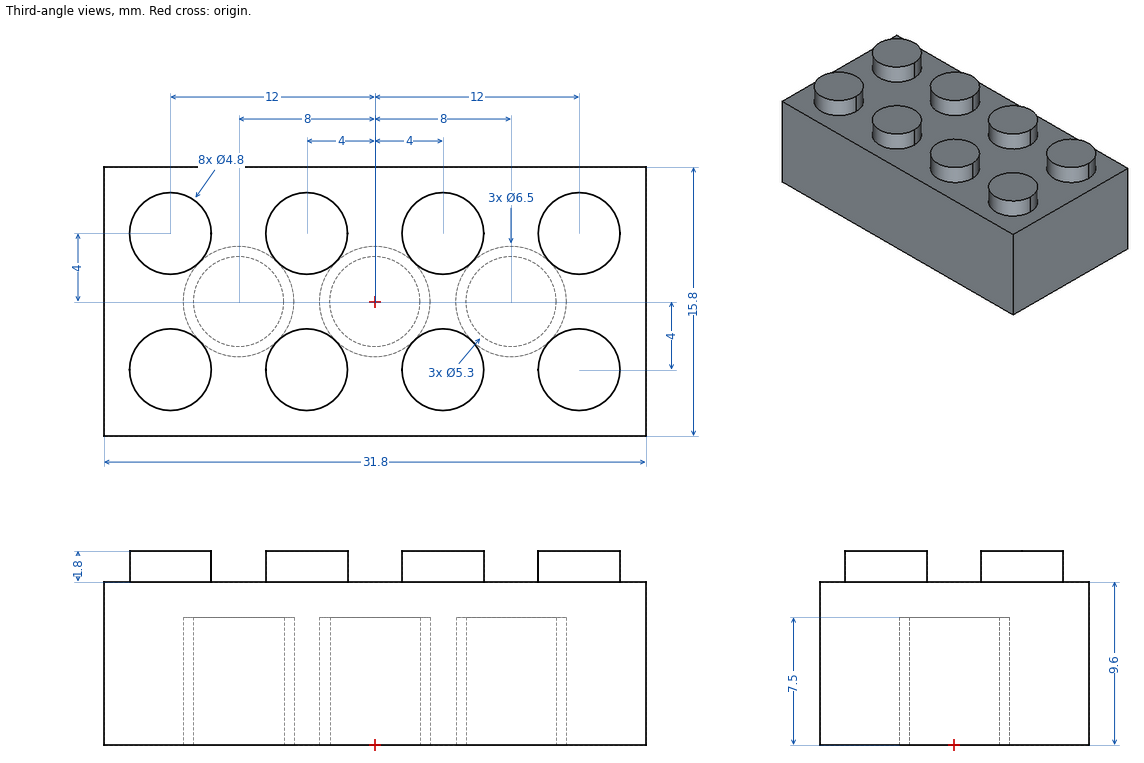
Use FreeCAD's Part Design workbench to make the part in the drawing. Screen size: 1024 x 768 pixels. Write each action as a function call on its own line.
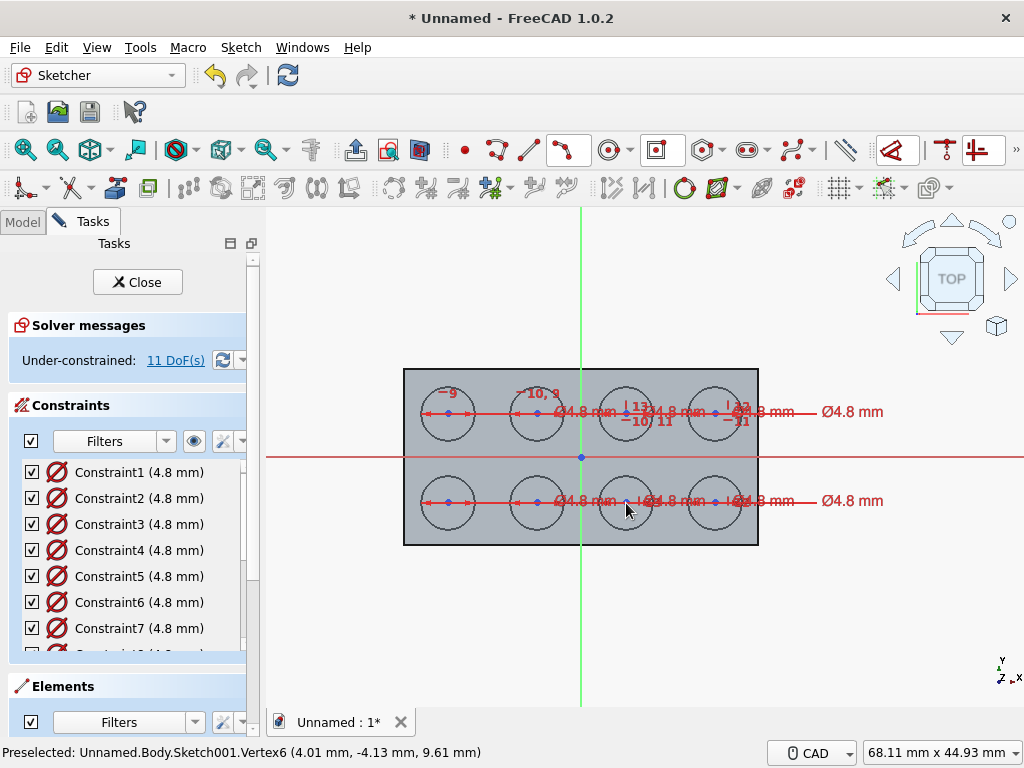
click(715, 503)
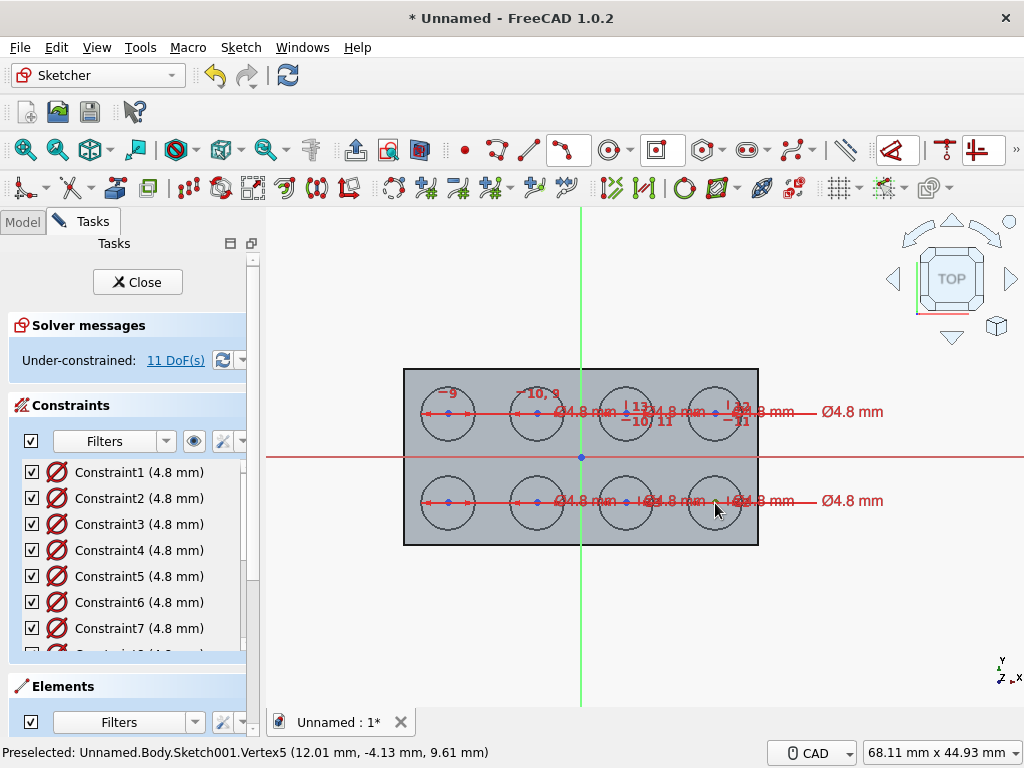
click(626, 503)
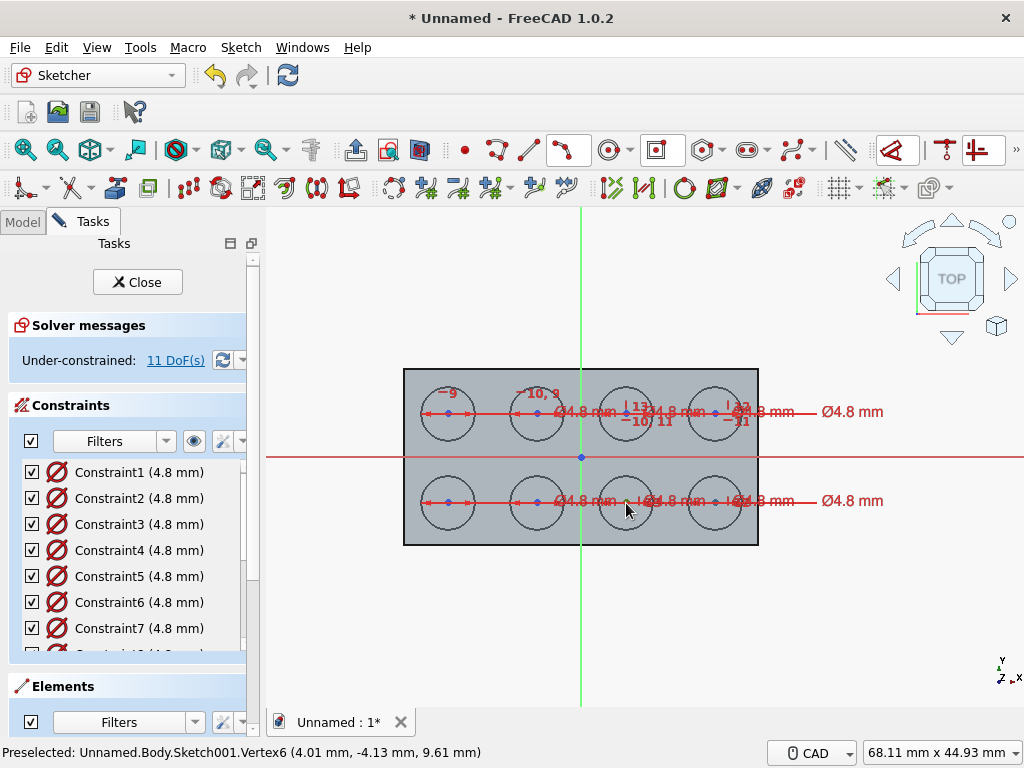
click(1000, 150)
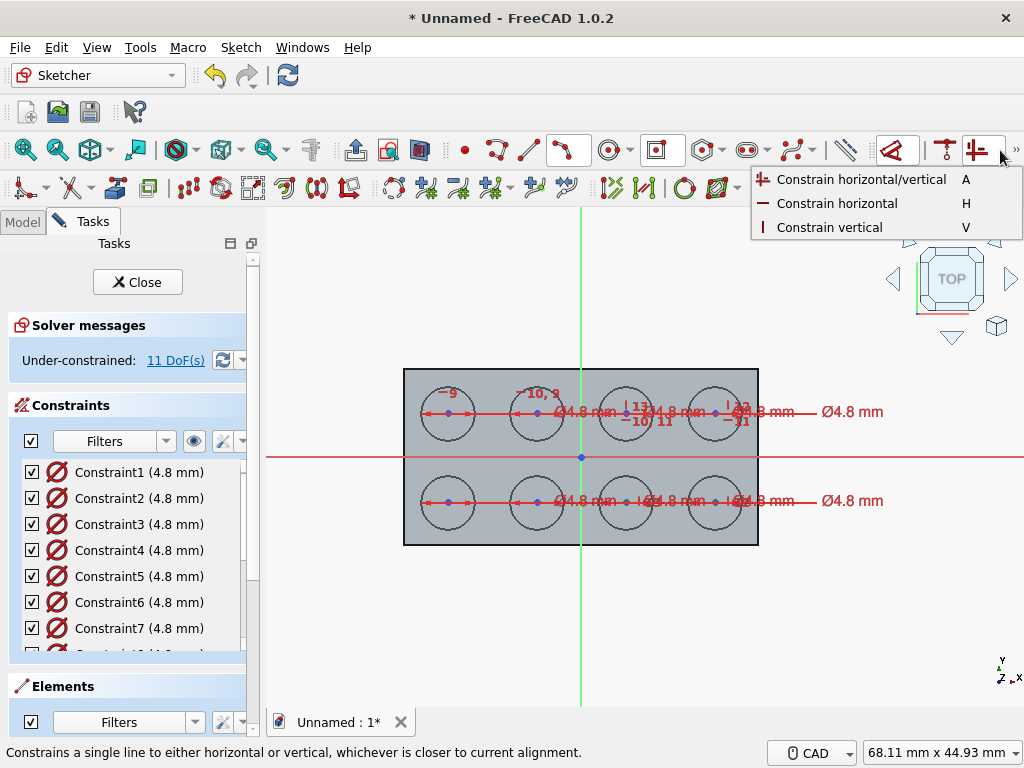
click(887, 203)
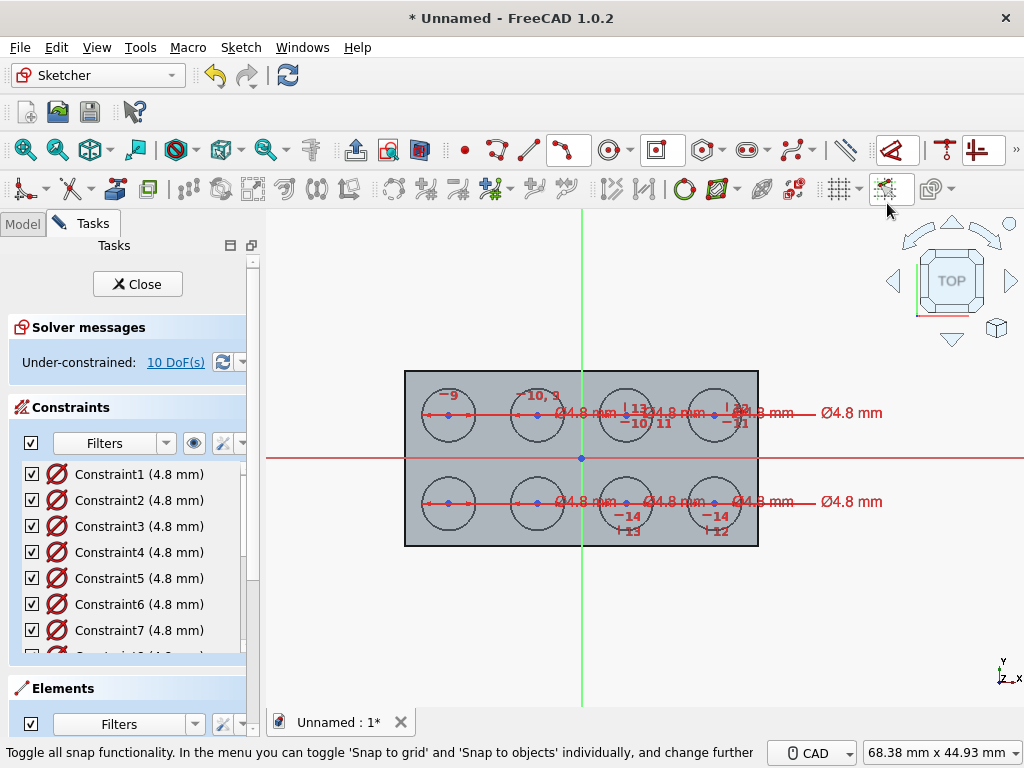
click(537, 415)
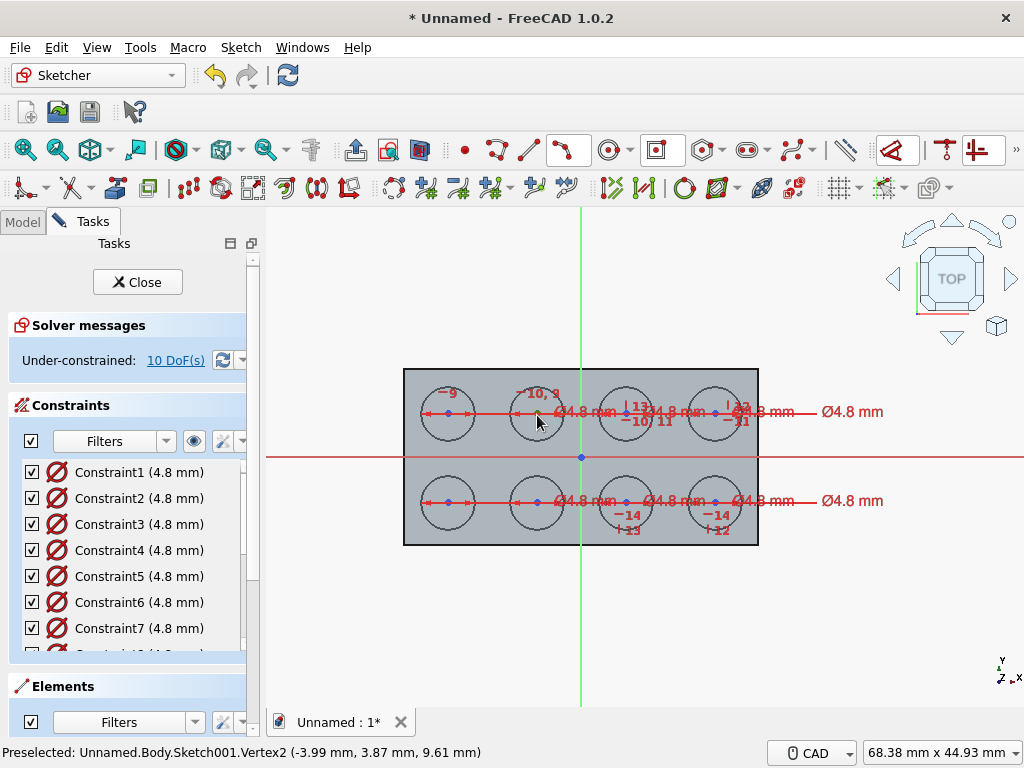
click(537, 503)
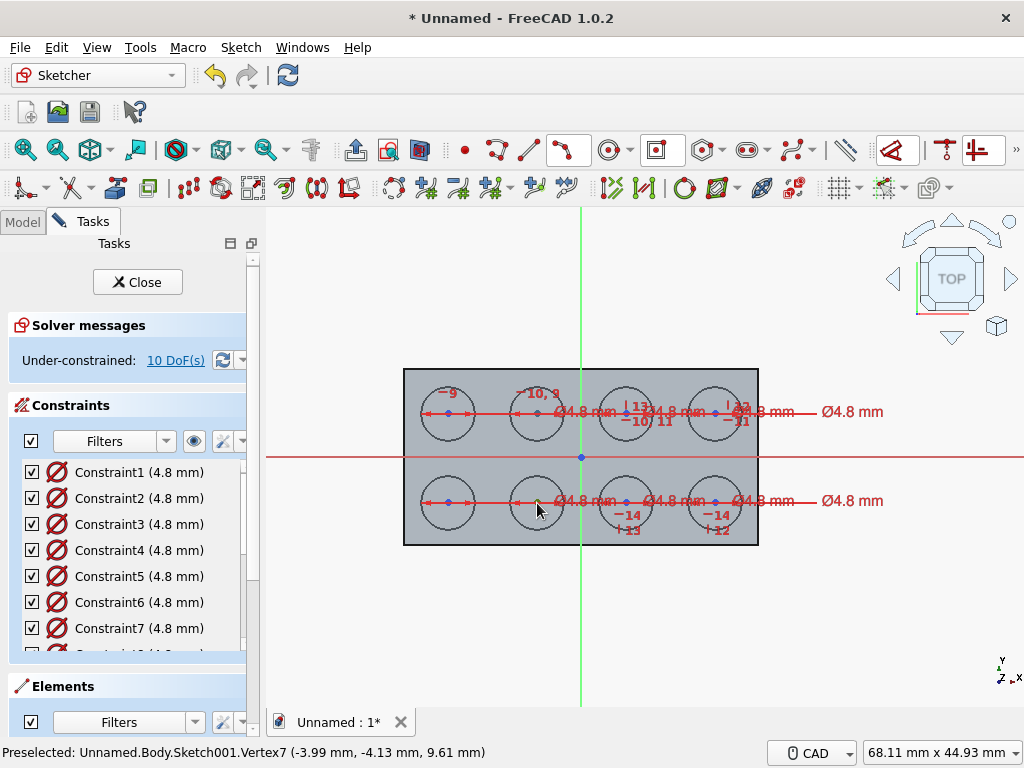
click(1000, 150)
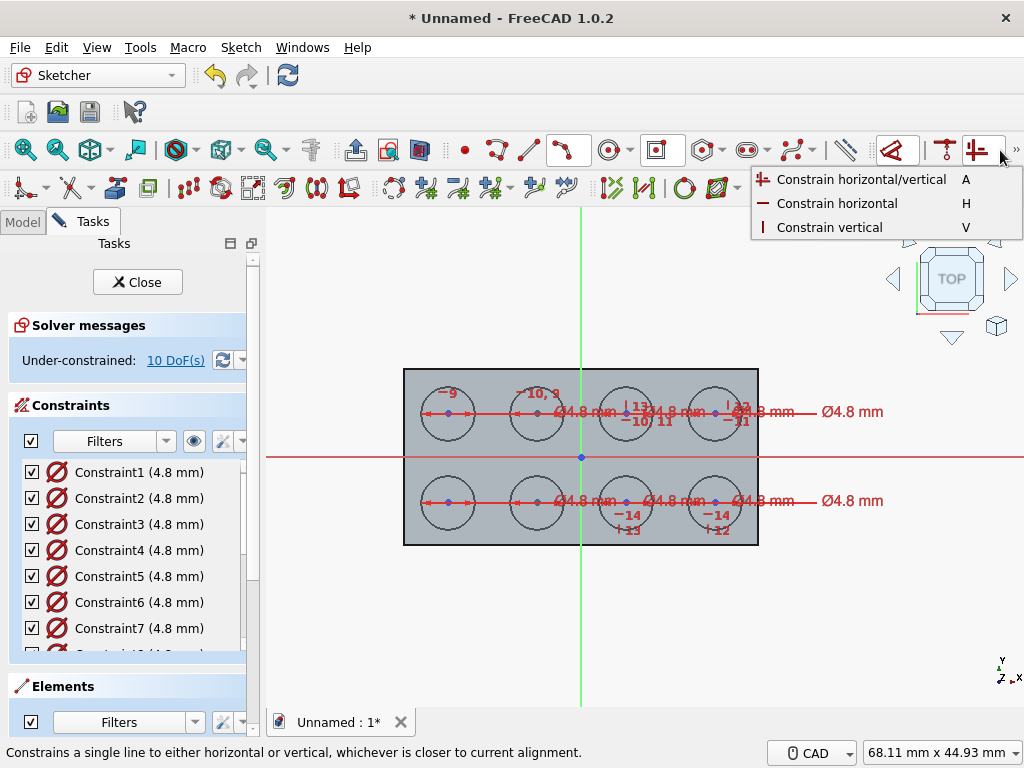
click(887, 227)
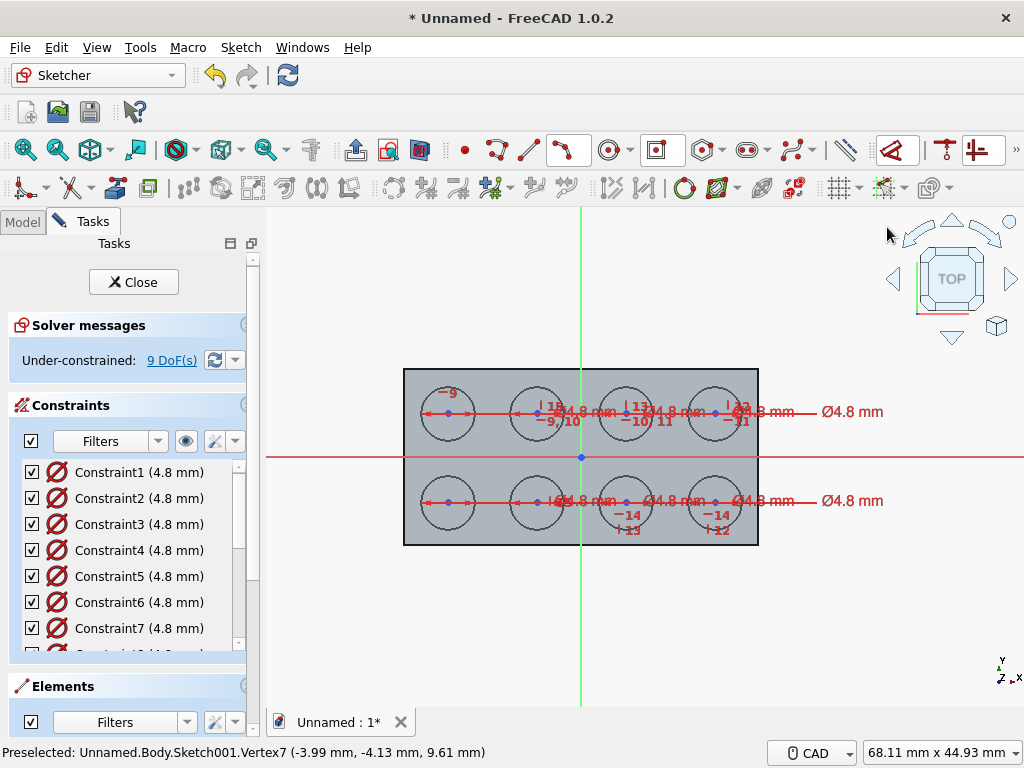
click(626, 503)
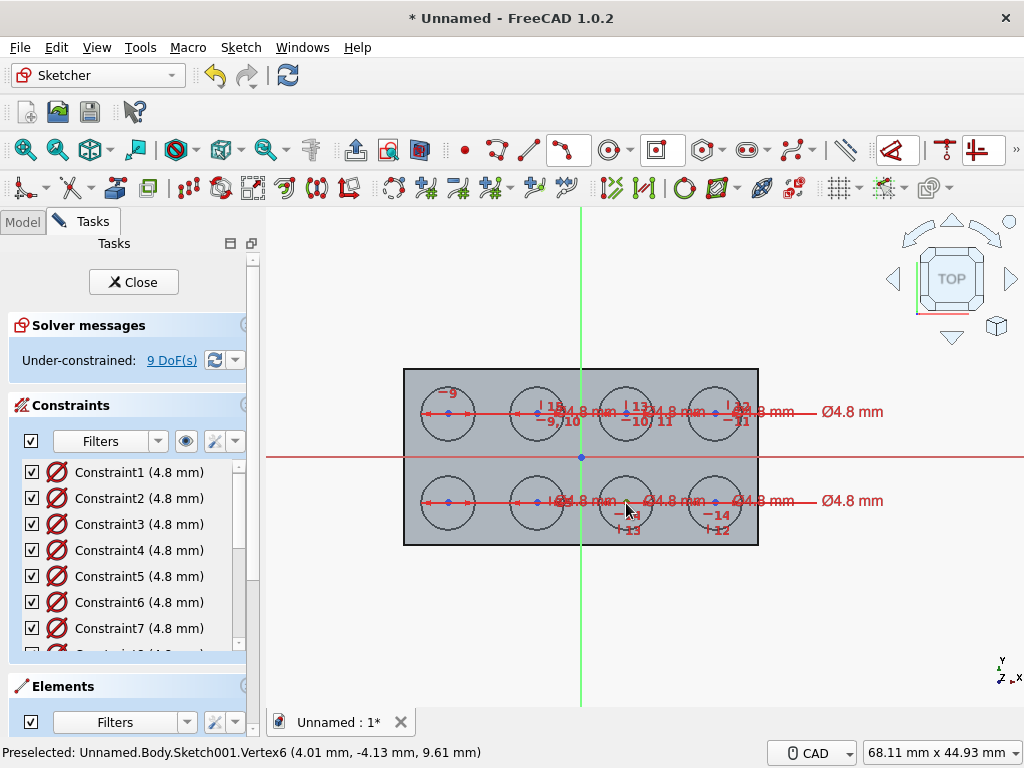
click(537, 503)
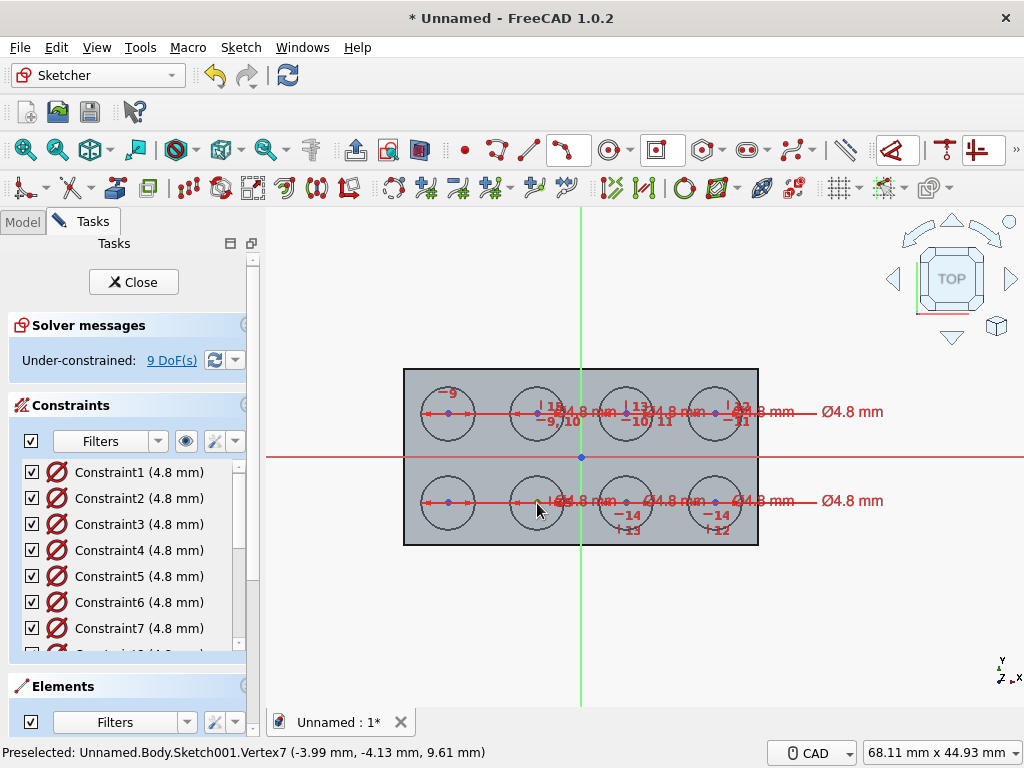
click(1000, 150)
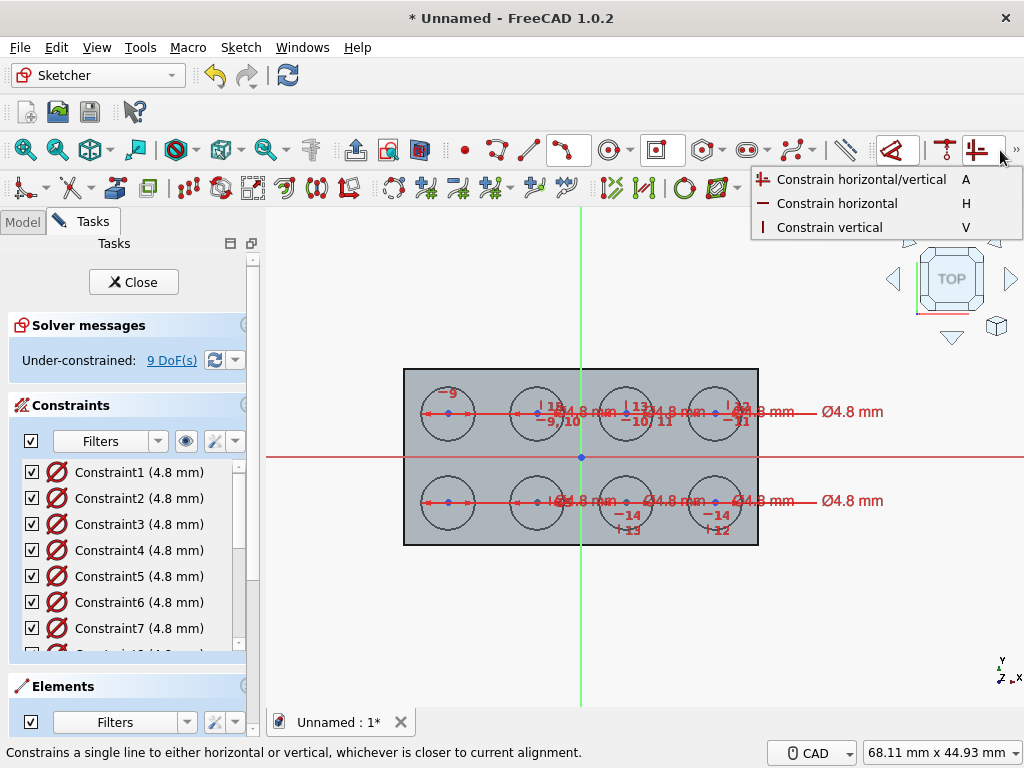
click(887, 203)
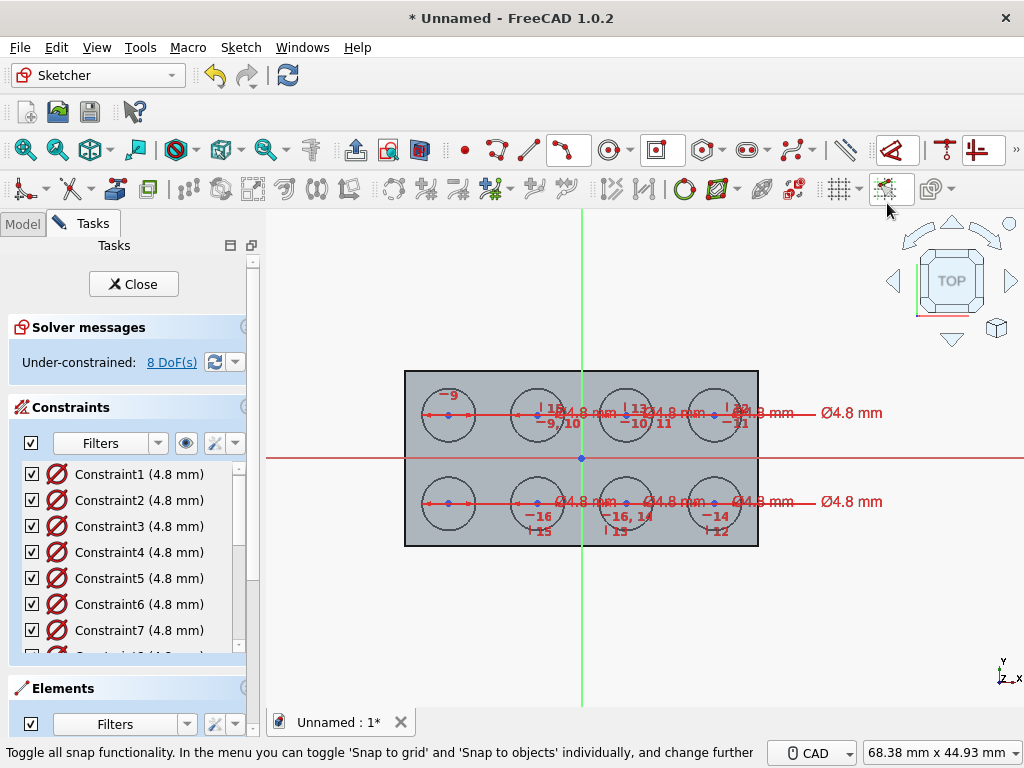
click(449, 415)